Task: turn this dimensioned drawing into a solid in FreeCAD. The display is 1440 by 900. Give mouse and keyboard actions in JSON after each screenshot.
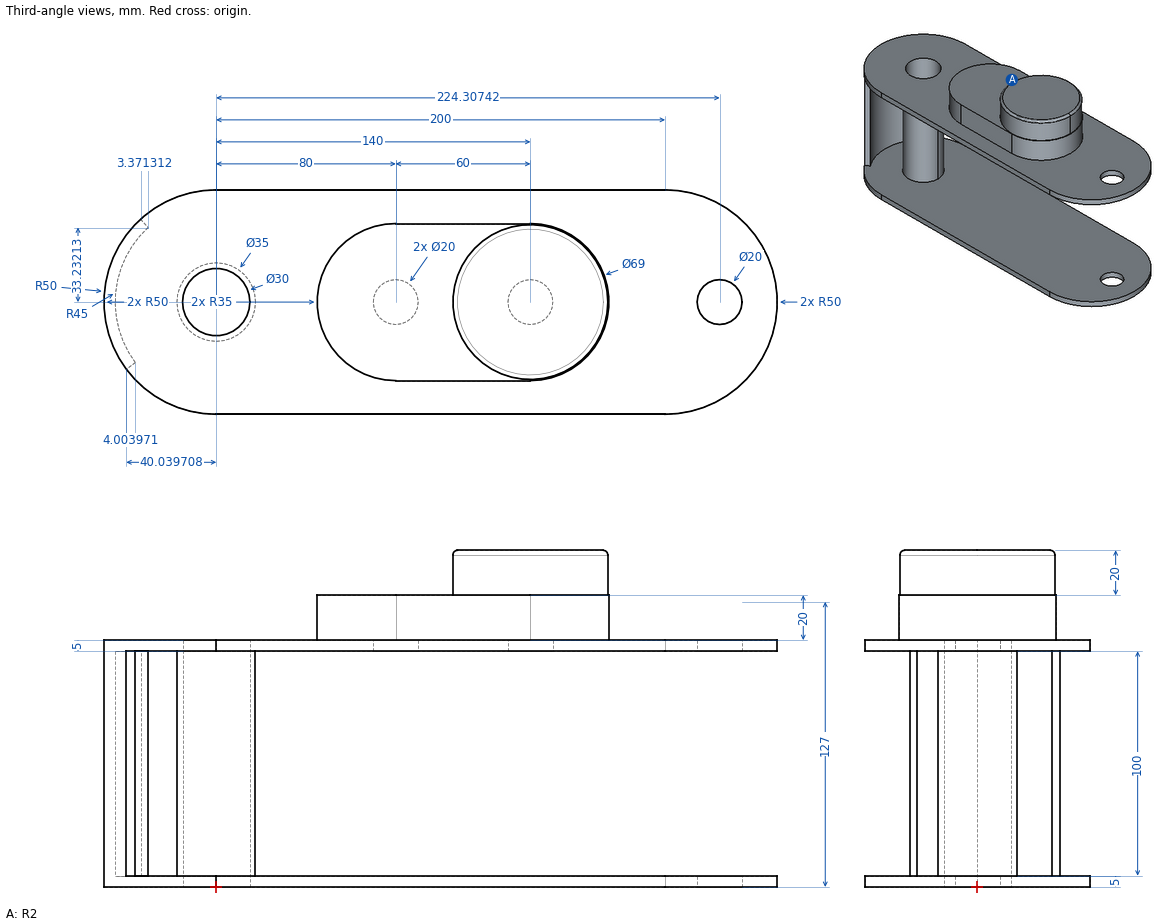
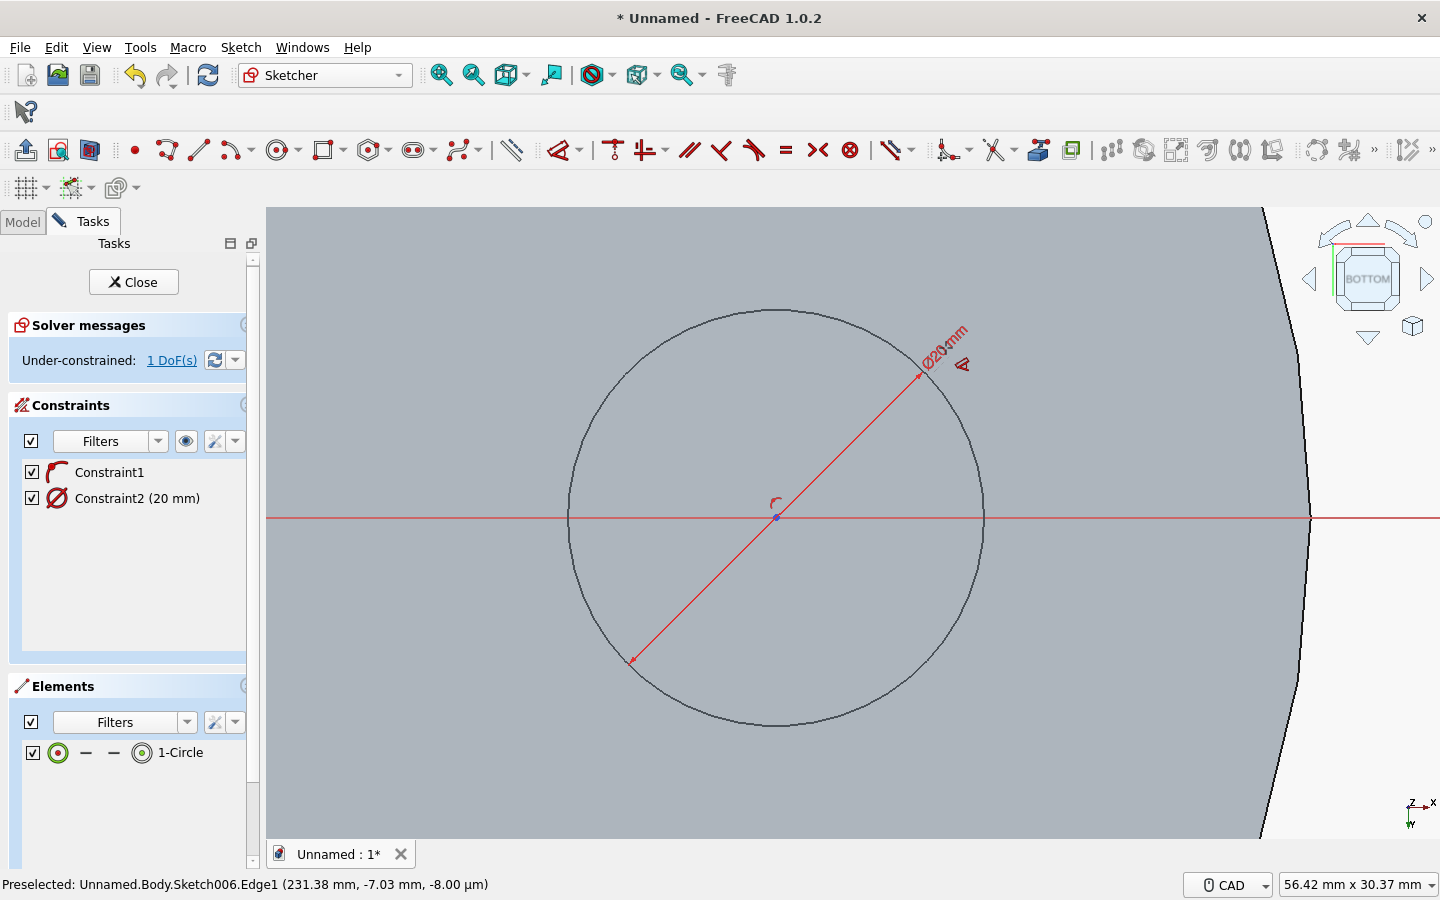
{"action": "left_click", "coordinate": [776, 518]}
{"action": "left_click", "coordinate": [535, 552]}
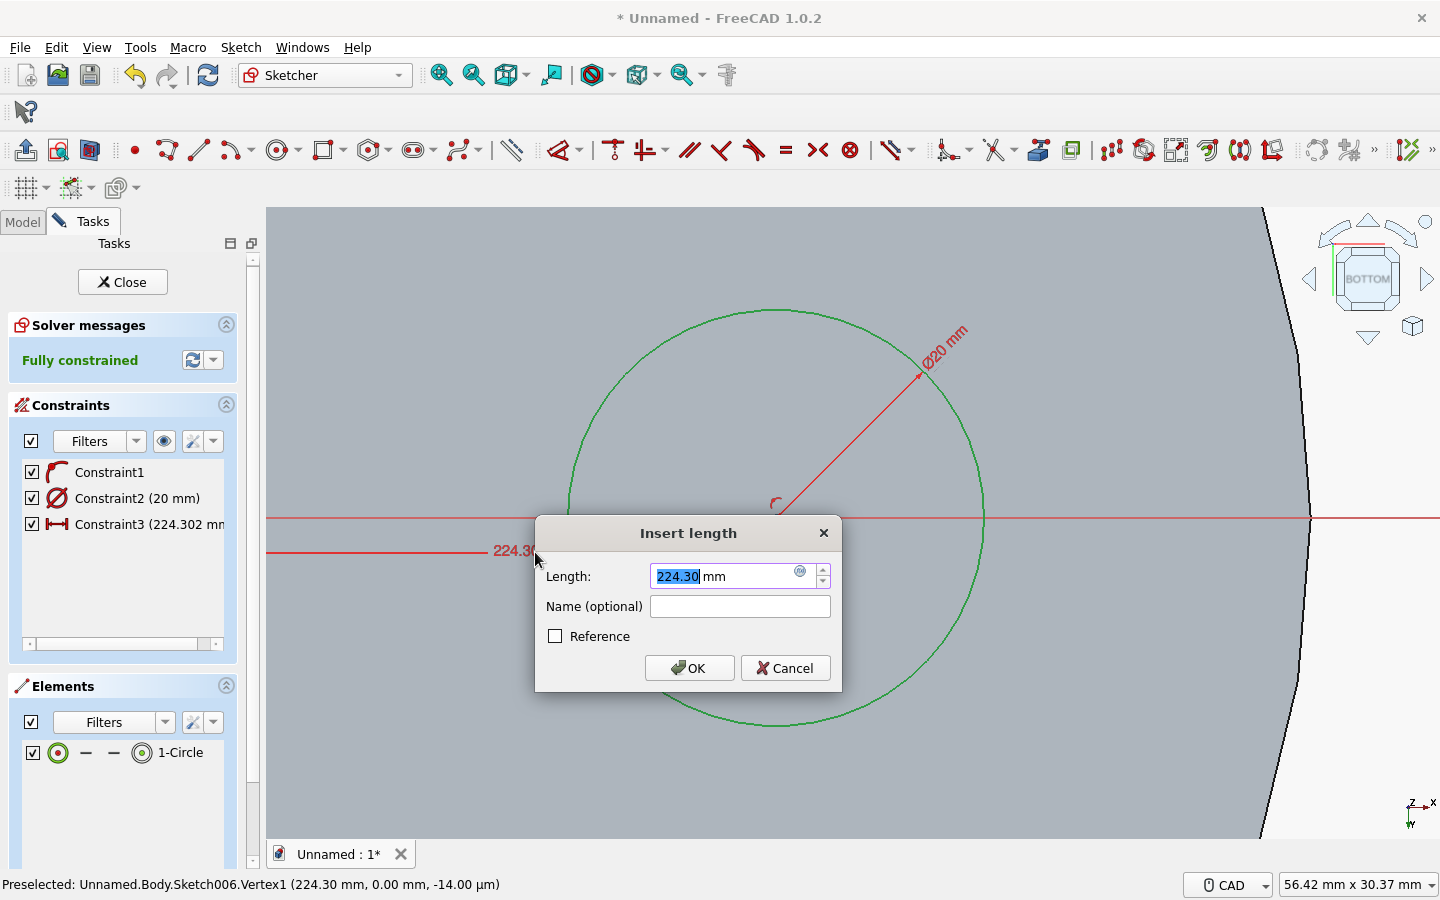
{"action": "type", "text": "224.30742"}
{"action": "key", "text": "Return"}
{"action": "key", "text": "Escape"}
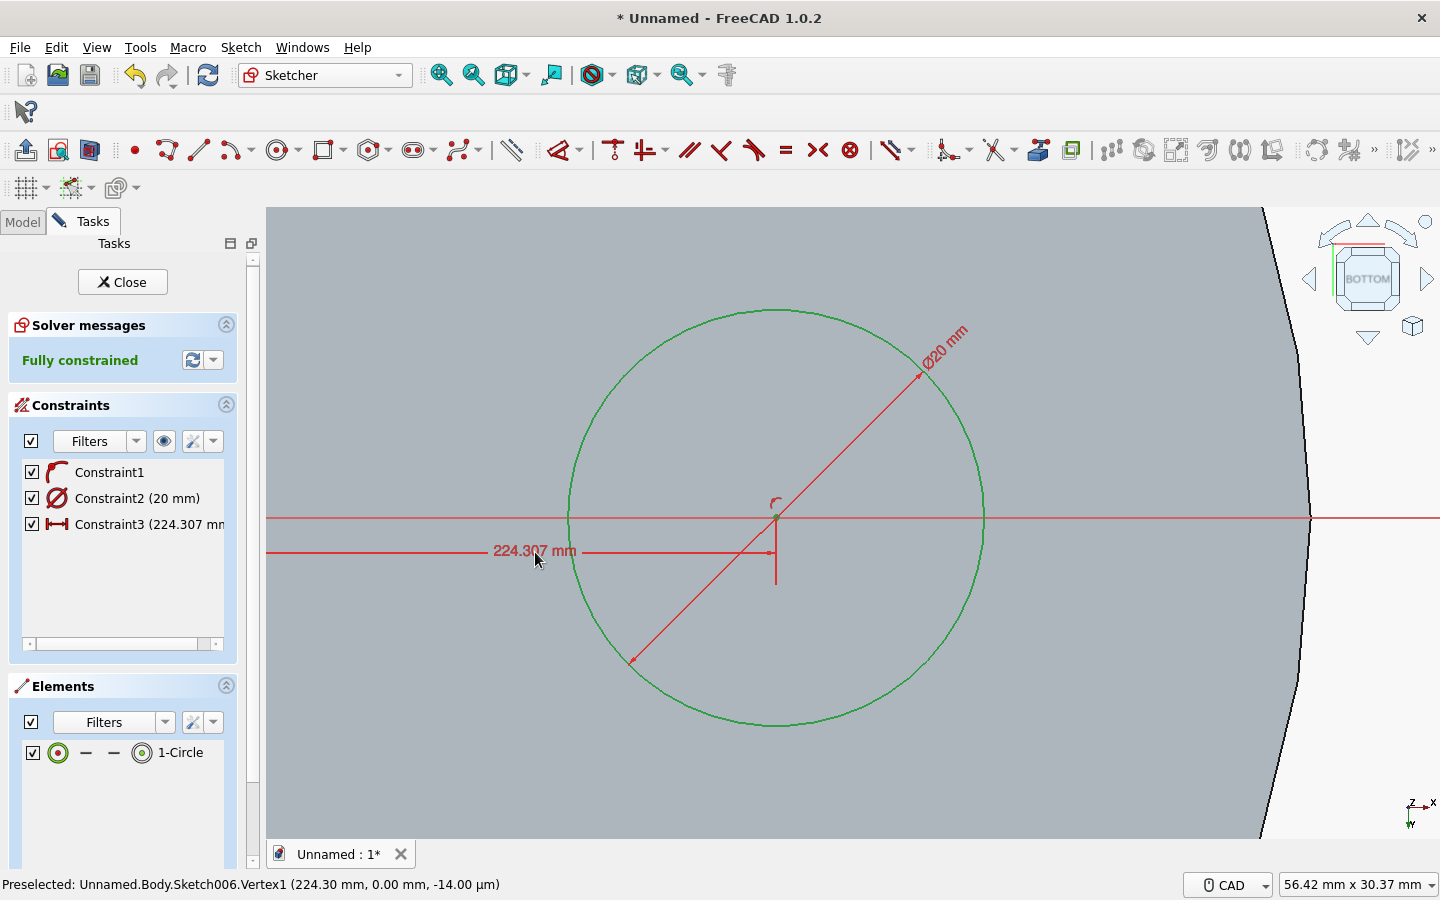
{"action": "left_click", "coordinate": [123, 282]}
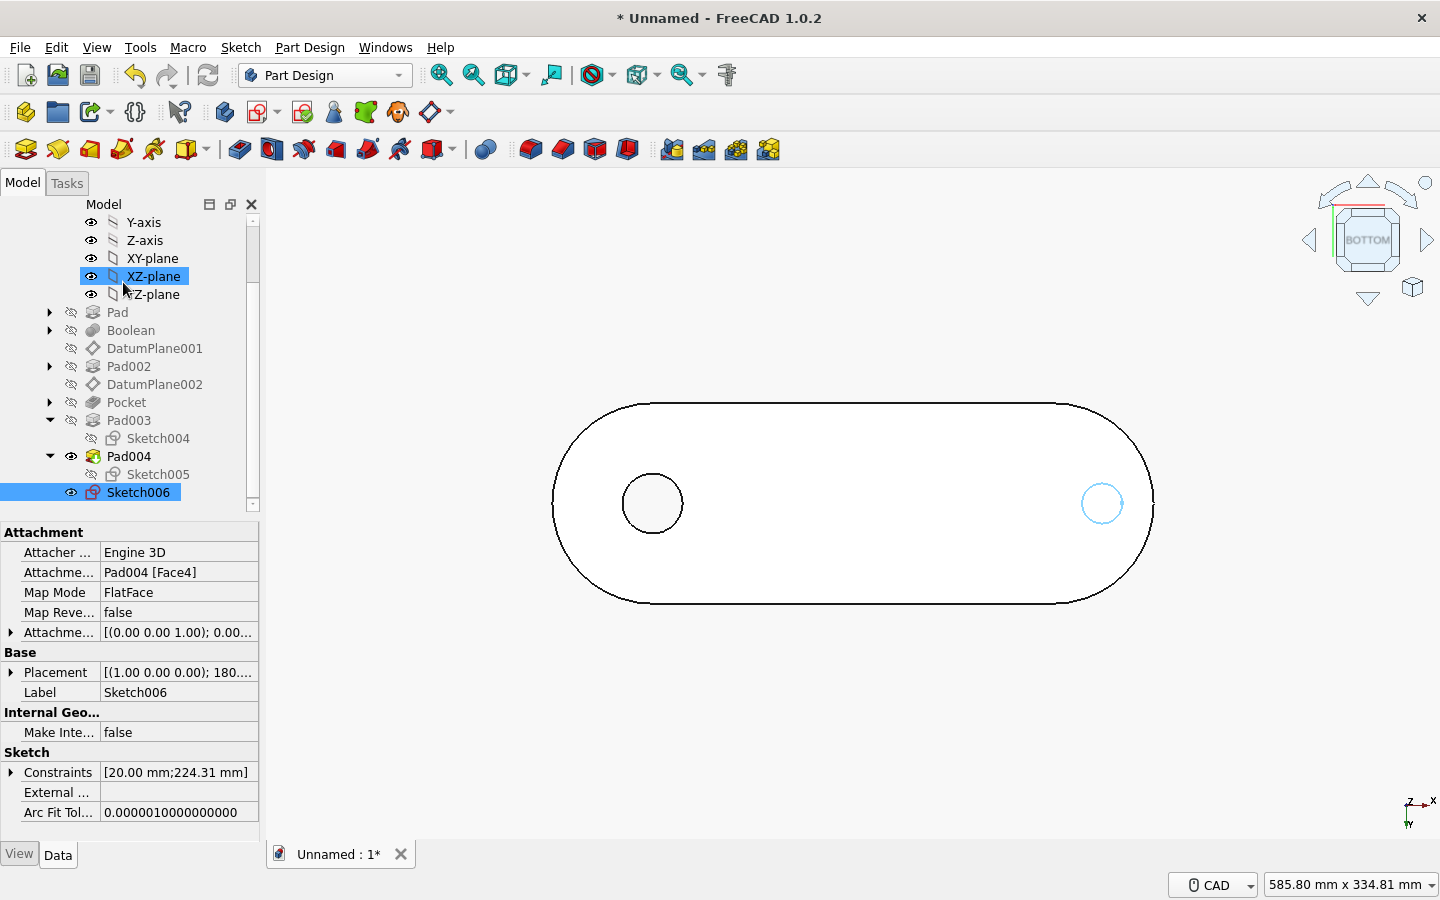
{"action": "left_click", "coordinate": [240, 150]}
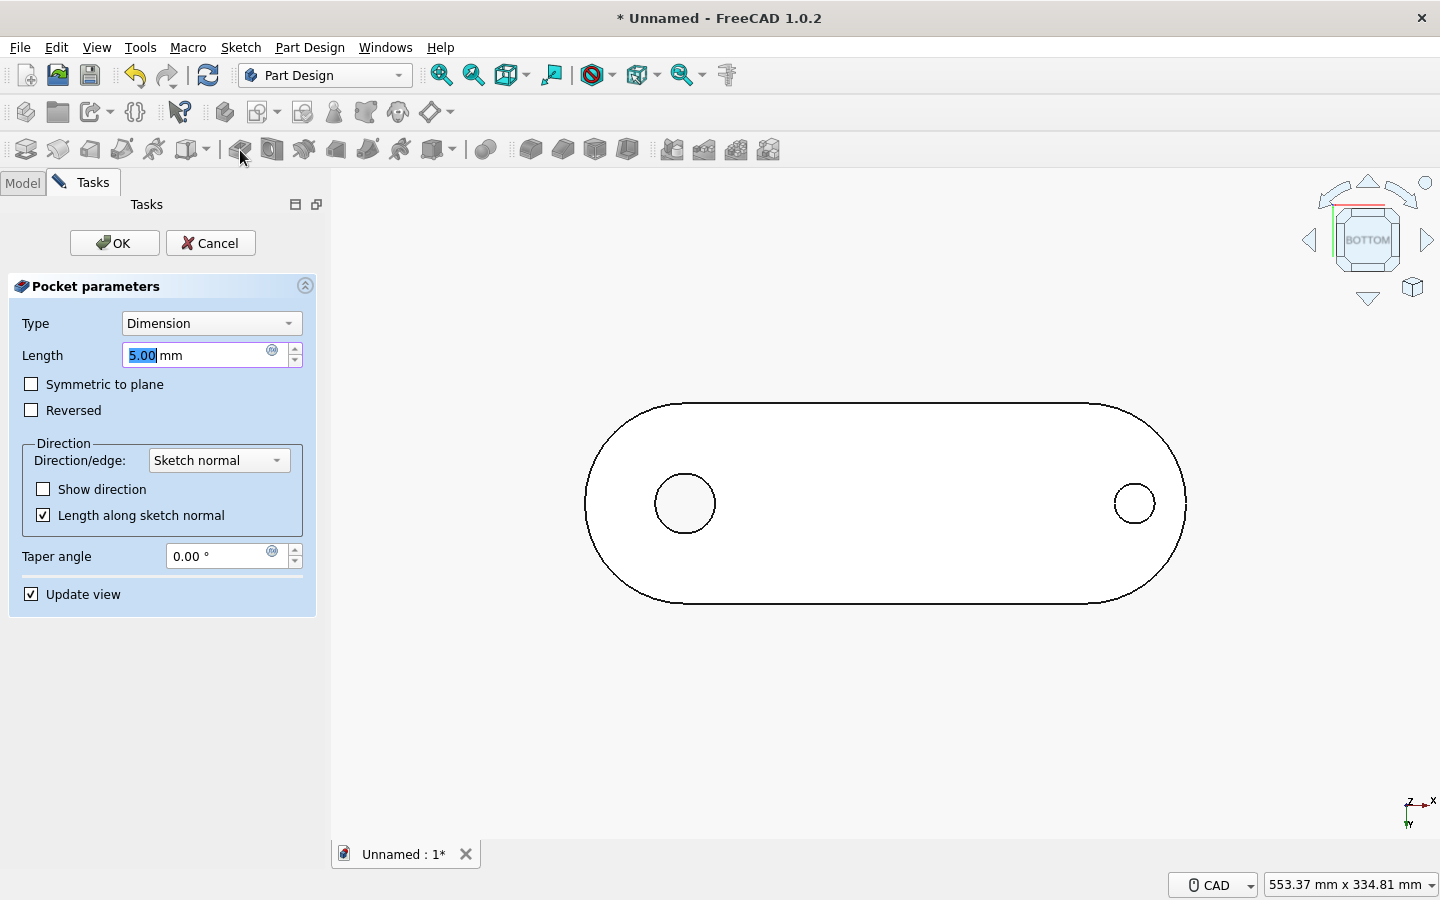
{"action": "type", "text": "127"}
{"action": "key", "text": "Tab"}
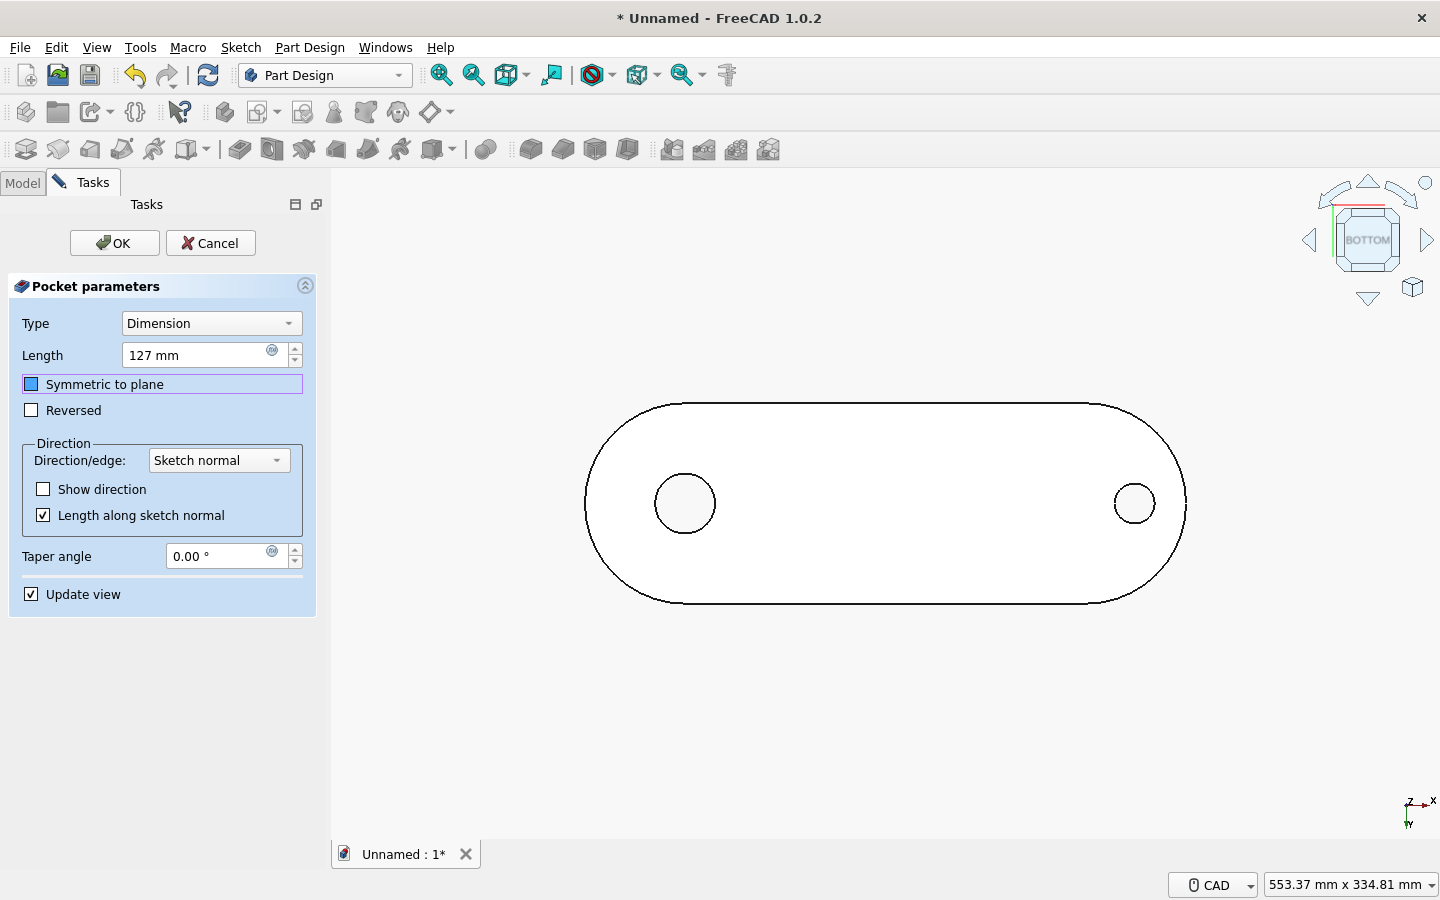
{"action": "left_click", "coordinate": [115, 243]}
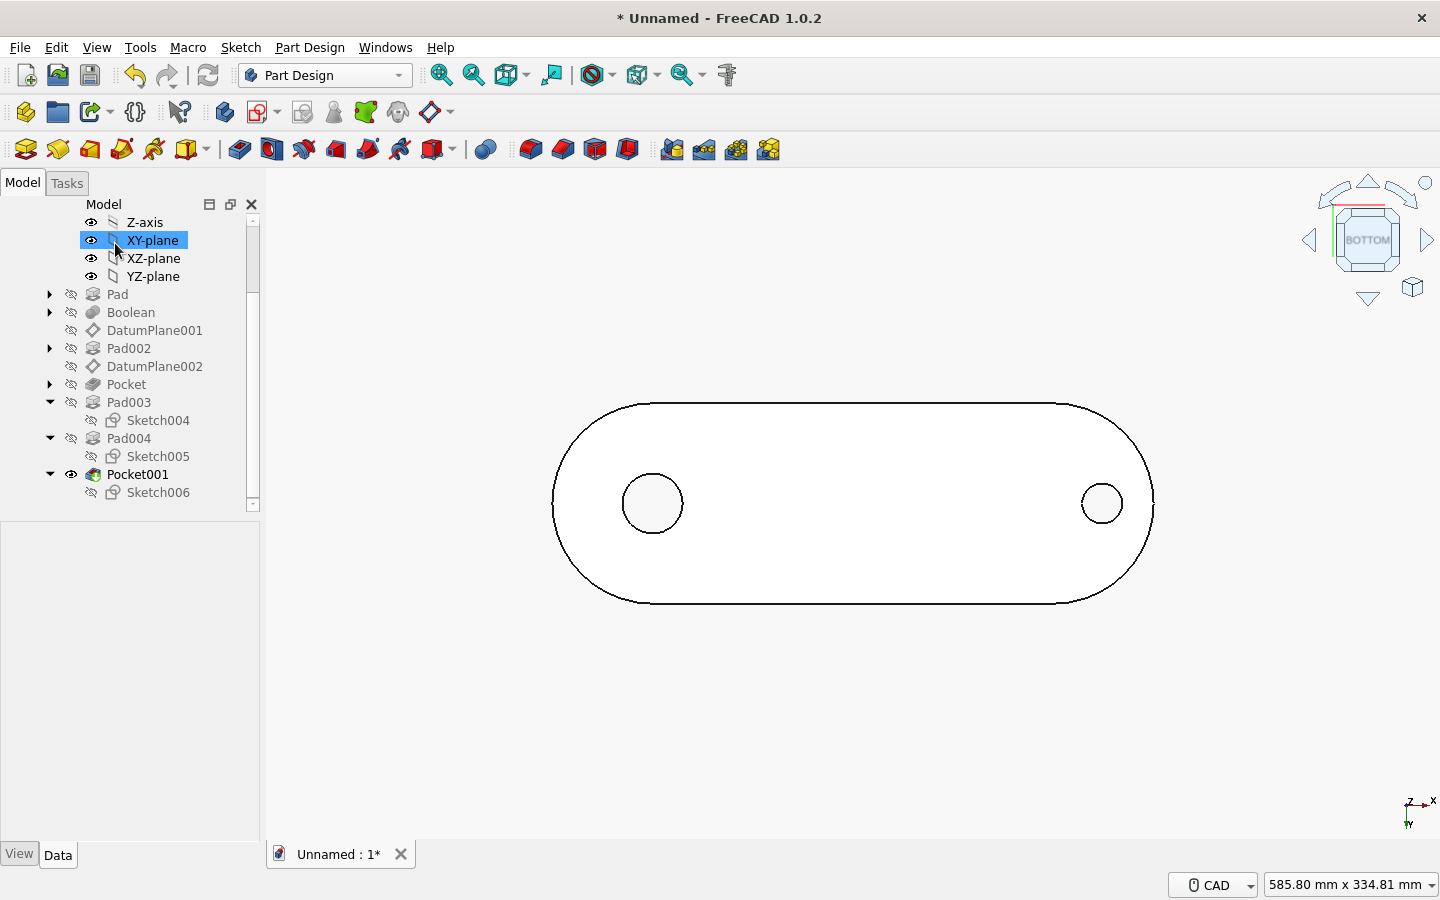
{"action": "scroll", "coordinate": [160, 362], "scroll_direction": "down", "scroll_amount": 3}